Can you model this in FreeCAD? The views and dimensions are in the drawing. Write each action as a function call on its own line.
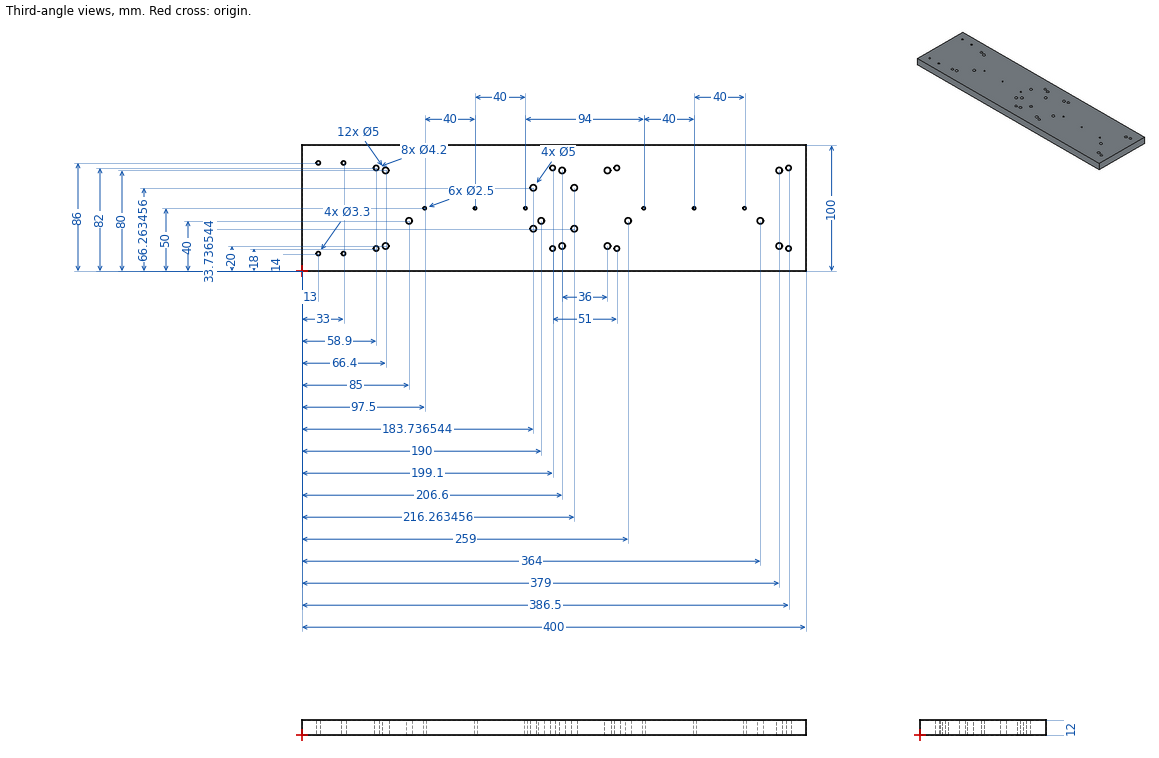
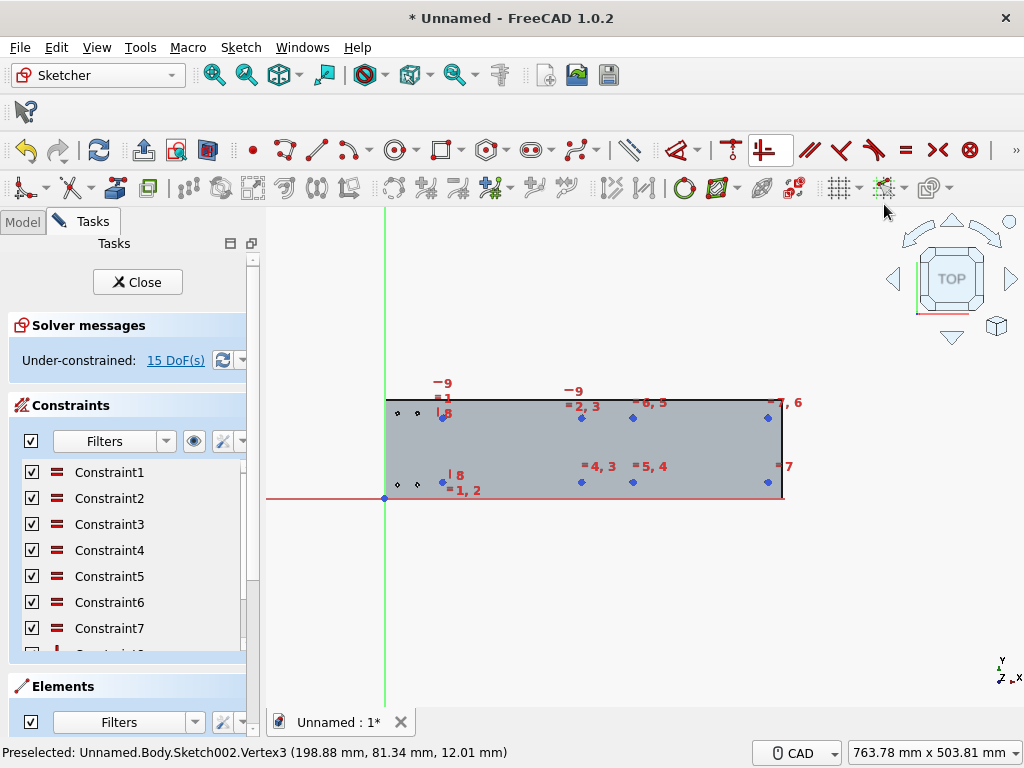
click(582, 418)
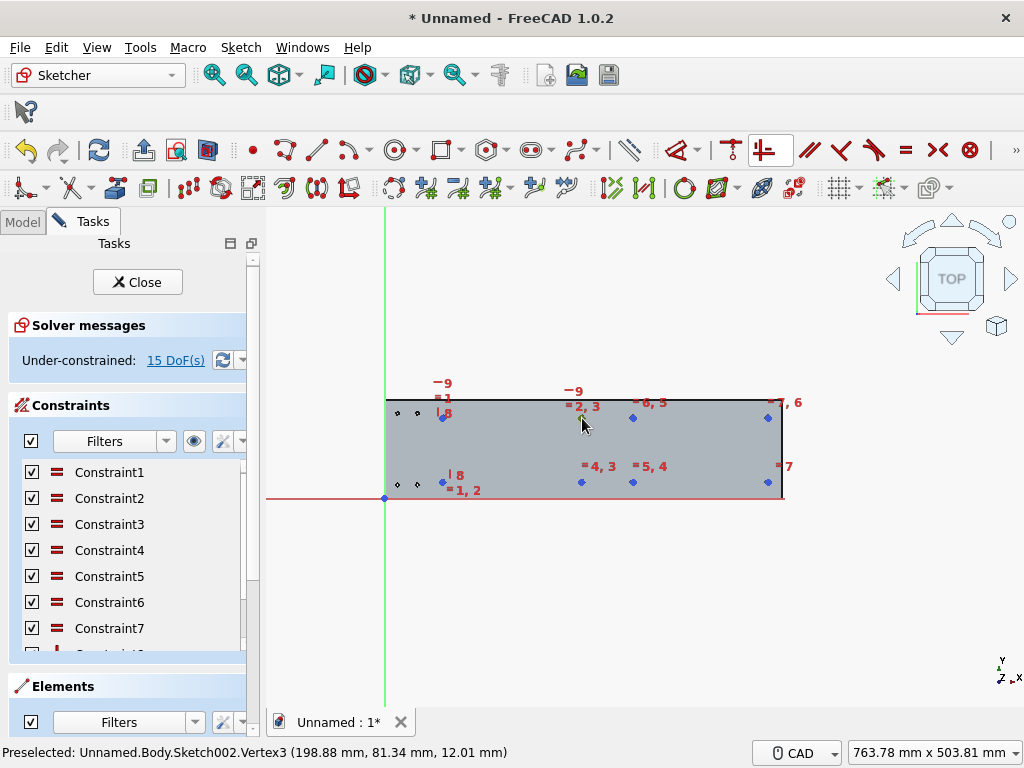
click(582, 482)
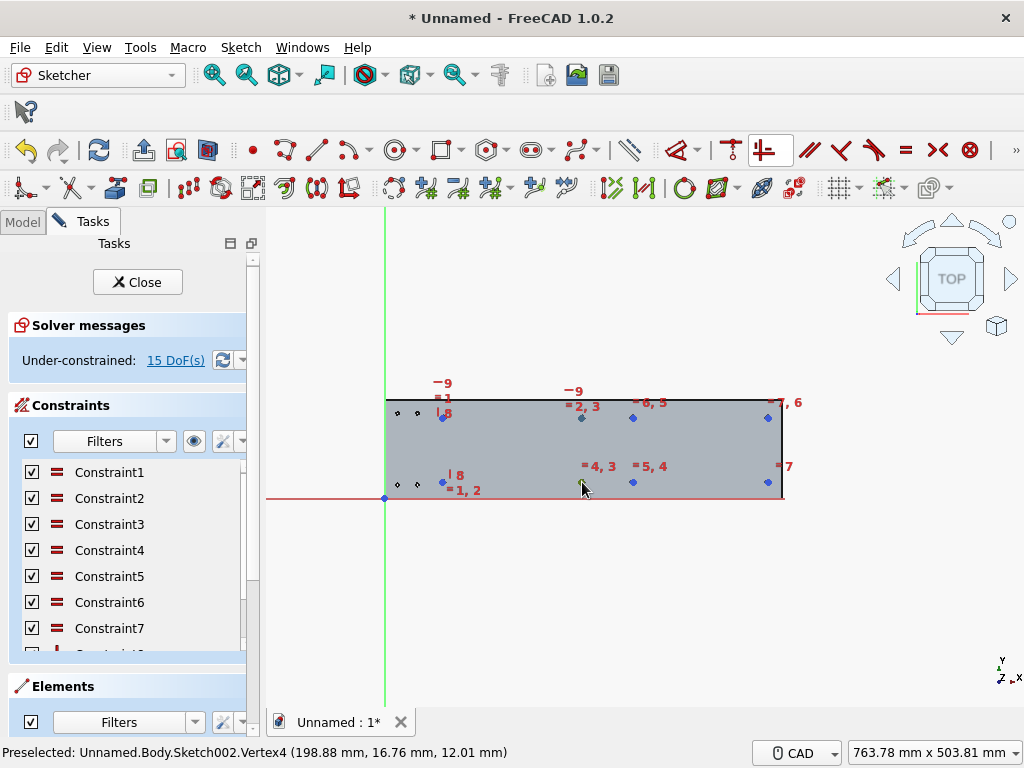
click(788, 150)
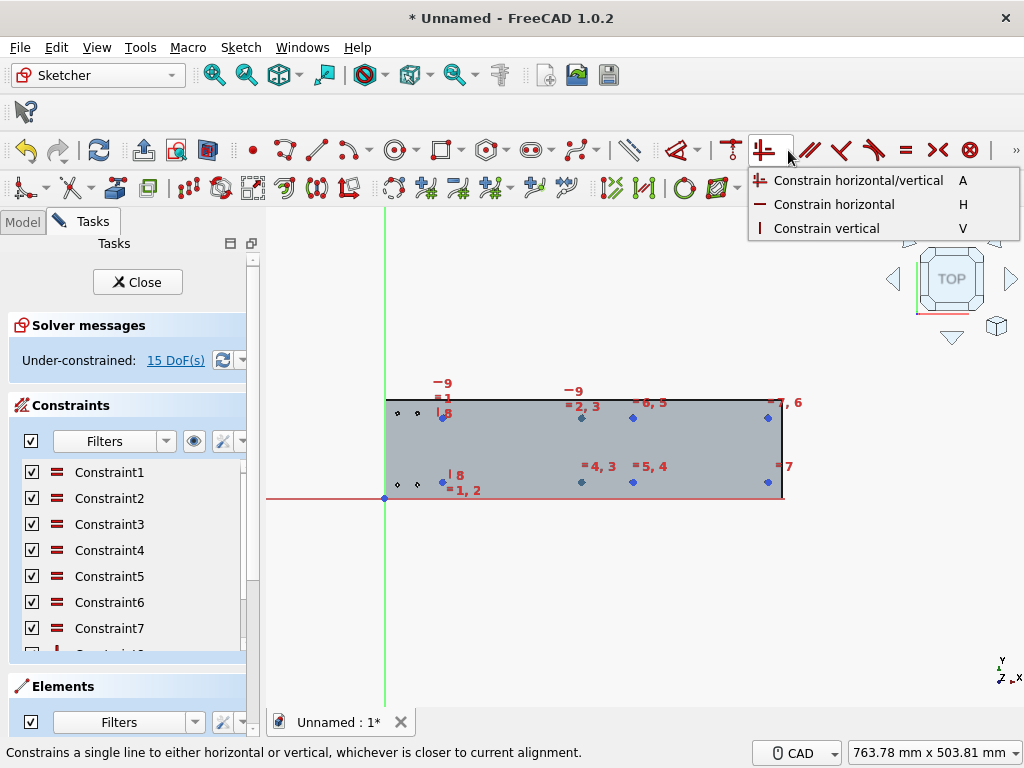
click(884, 228)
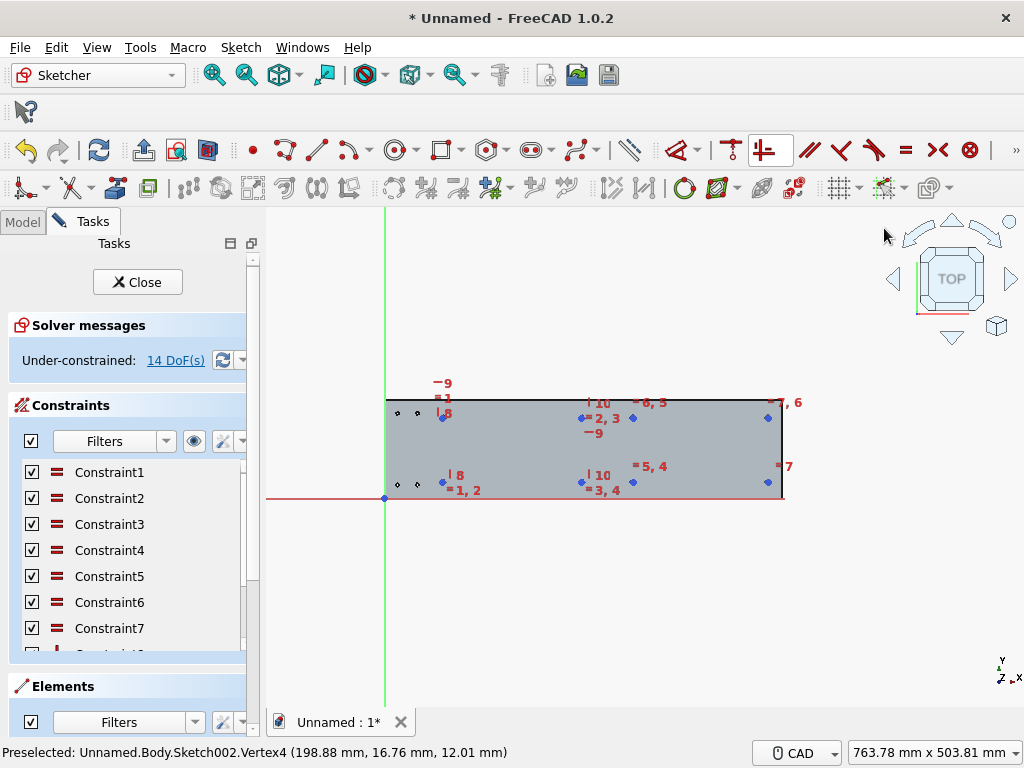
click(443, 482)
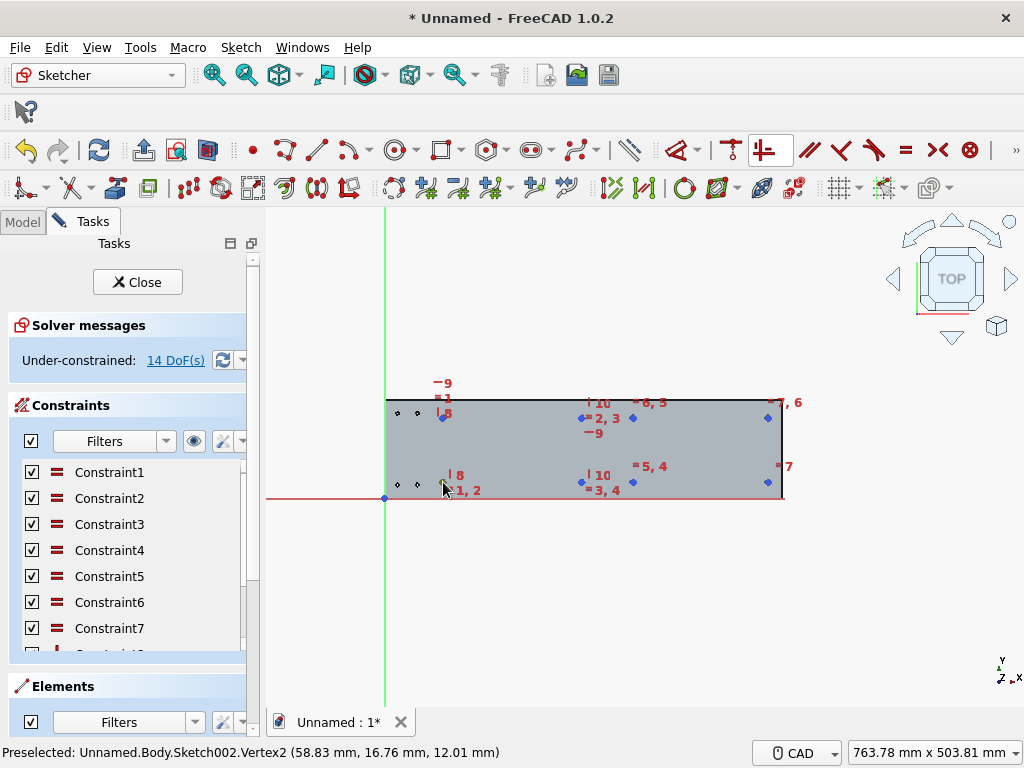
click(582, 482)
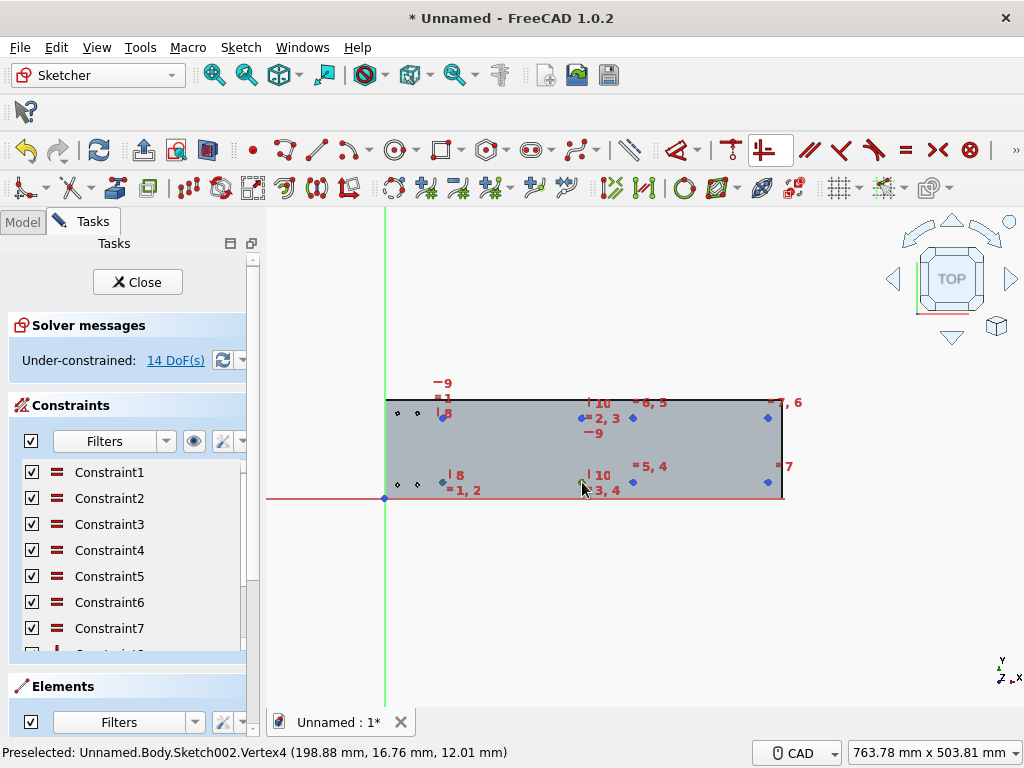
click(788, 150)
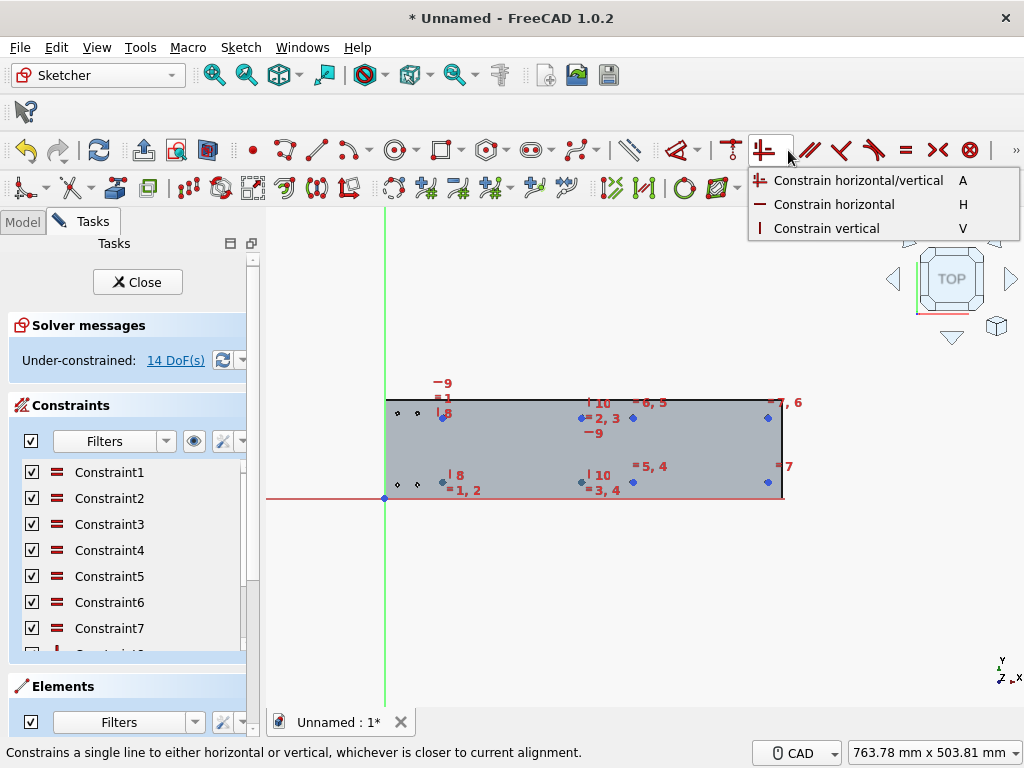
click(884, 204)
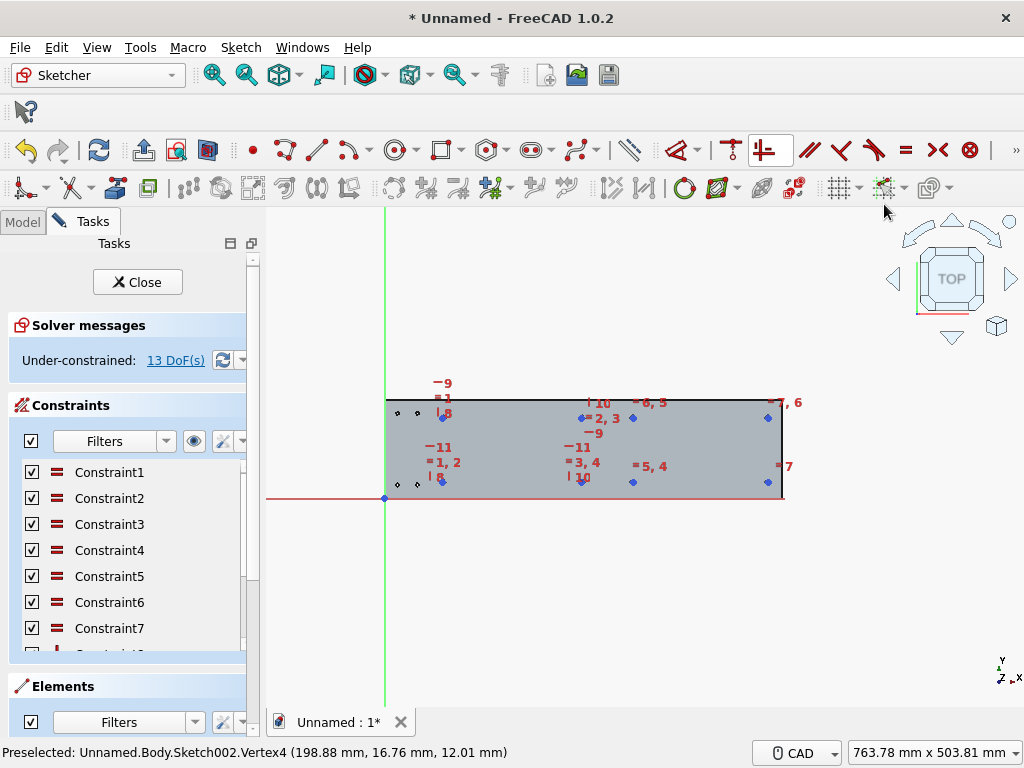
click(580, 484)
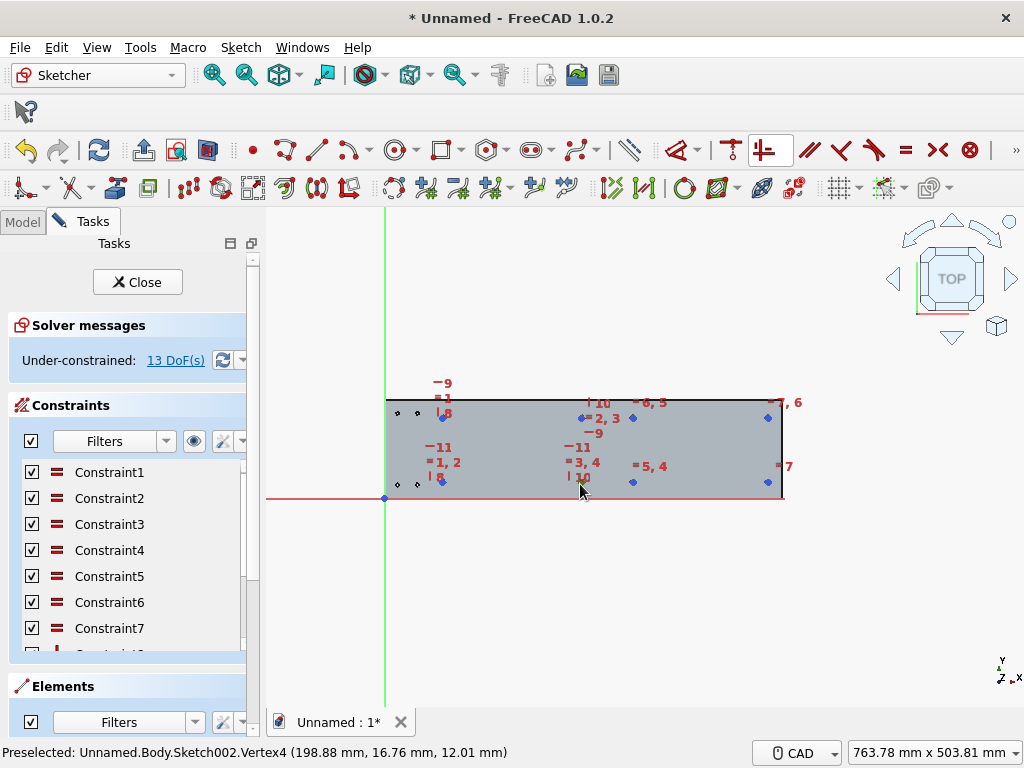
click(633, 482)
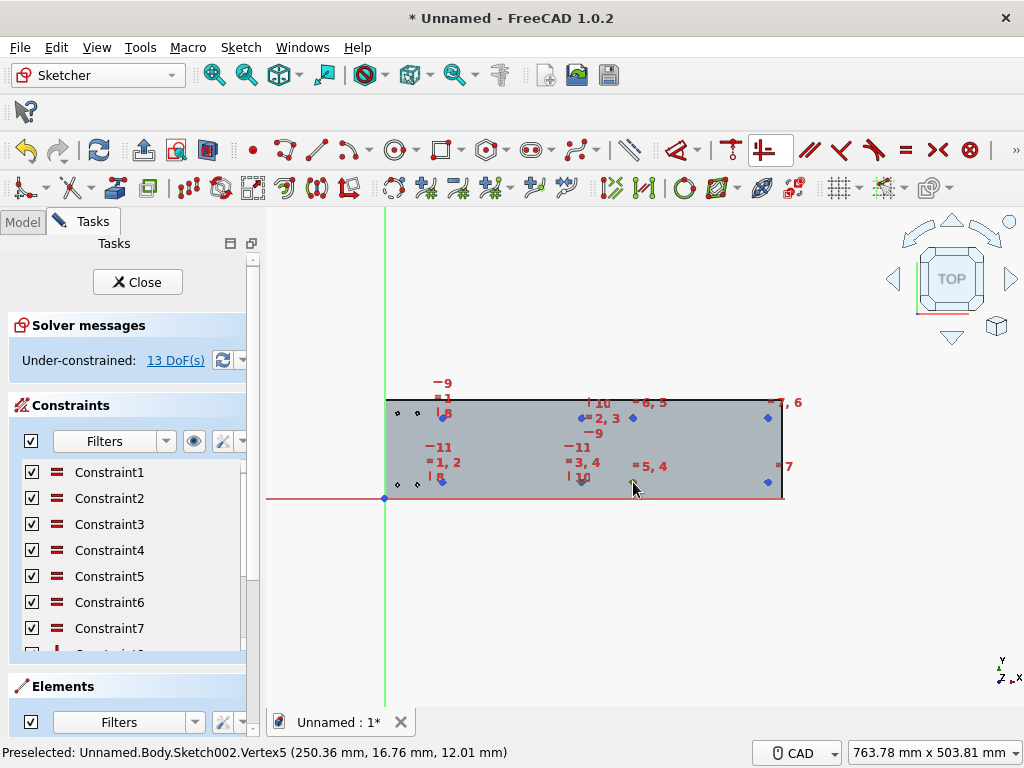
click(788, 150)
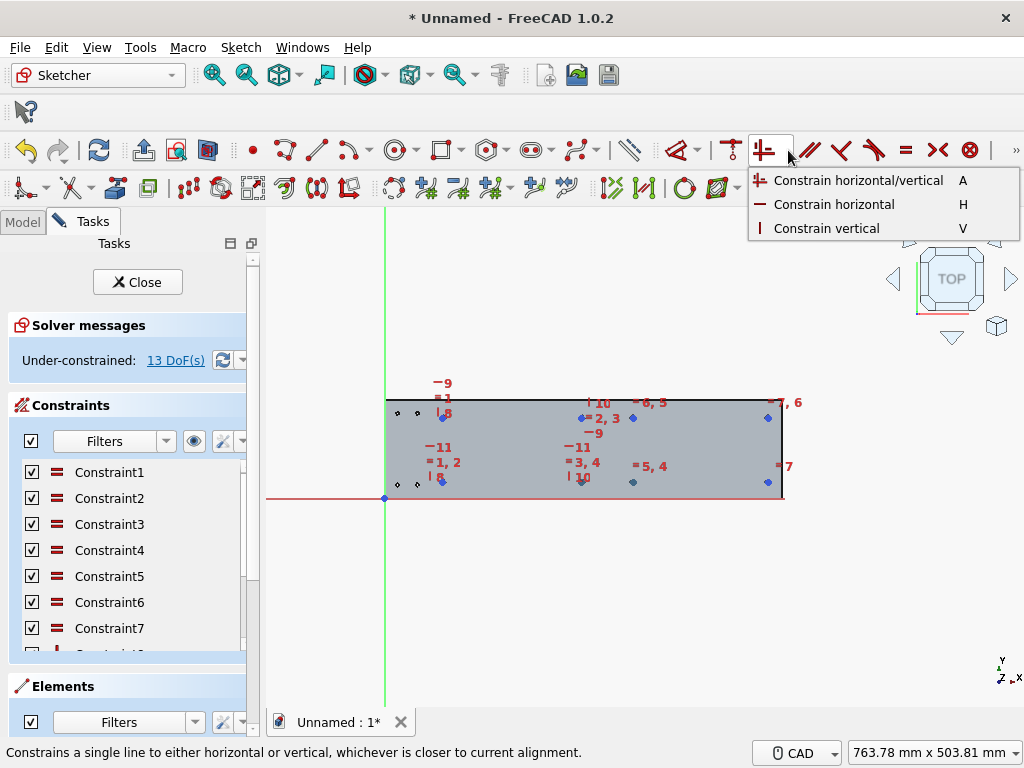
click(884, 204)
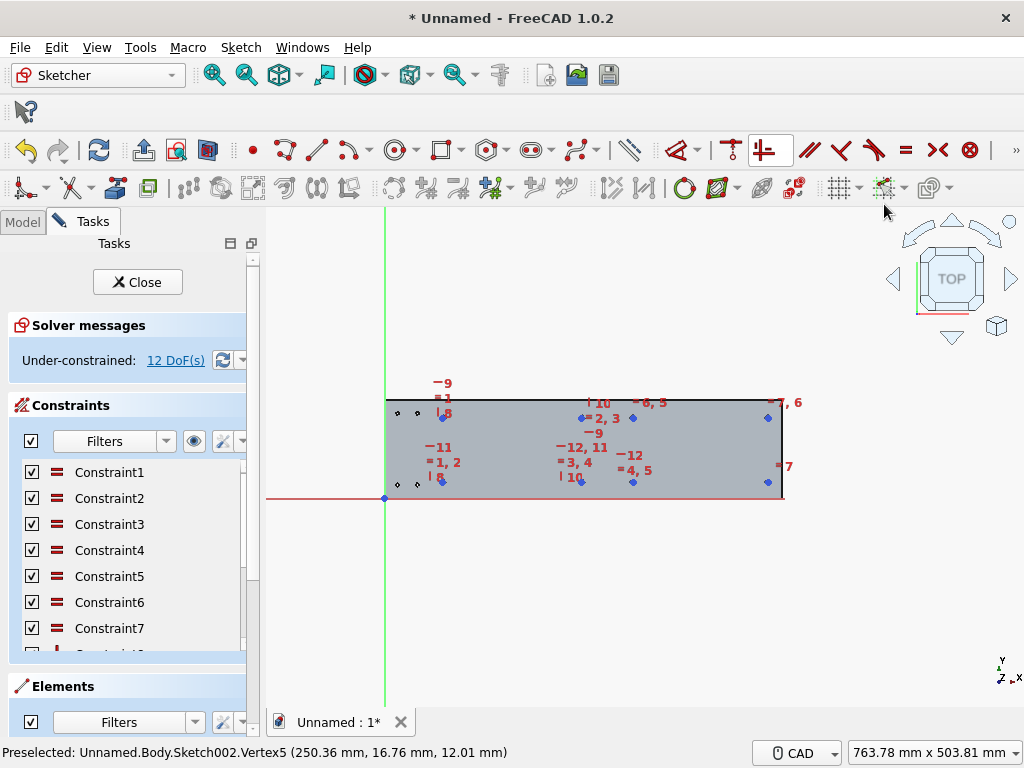
click(633, 482)